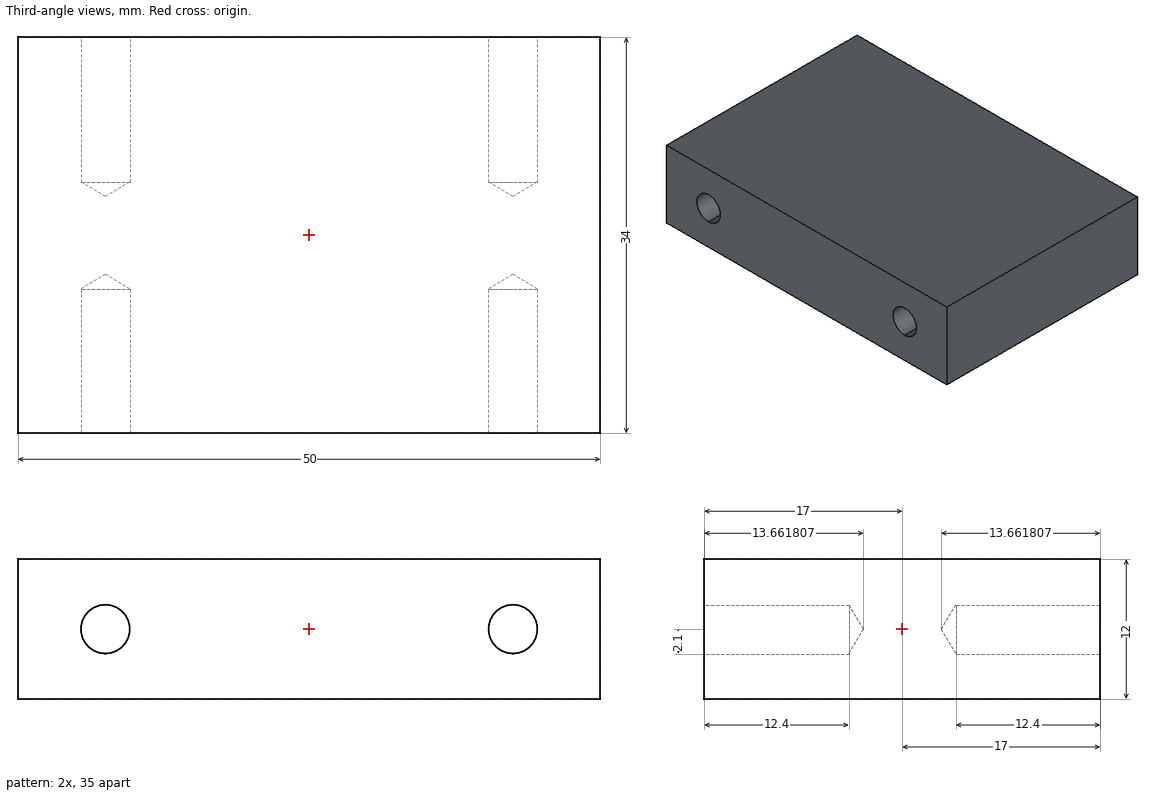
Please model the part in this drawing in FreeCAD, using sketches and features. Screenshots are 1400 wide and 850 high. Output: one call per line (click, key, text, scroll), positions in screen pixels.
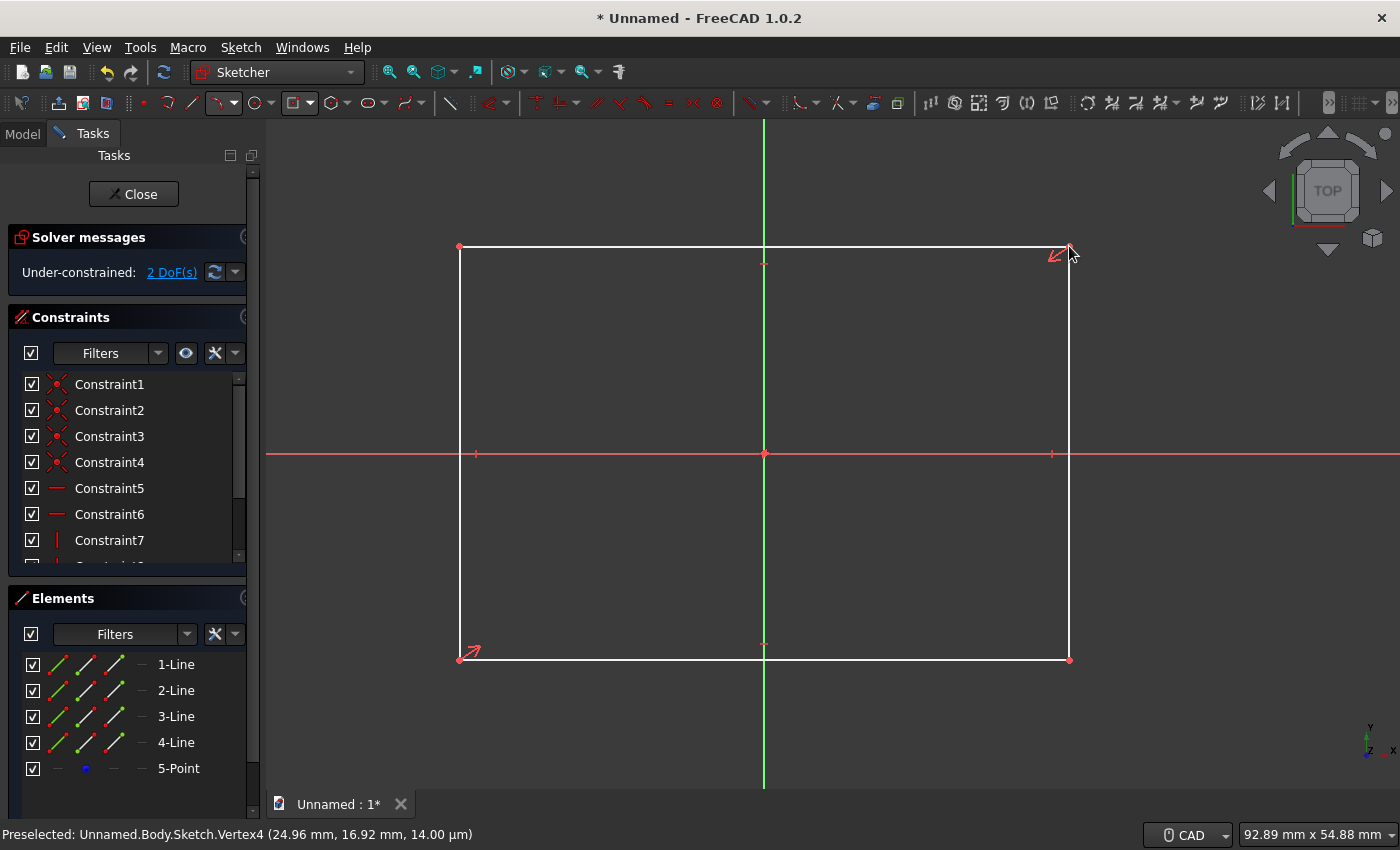
click(642, 660)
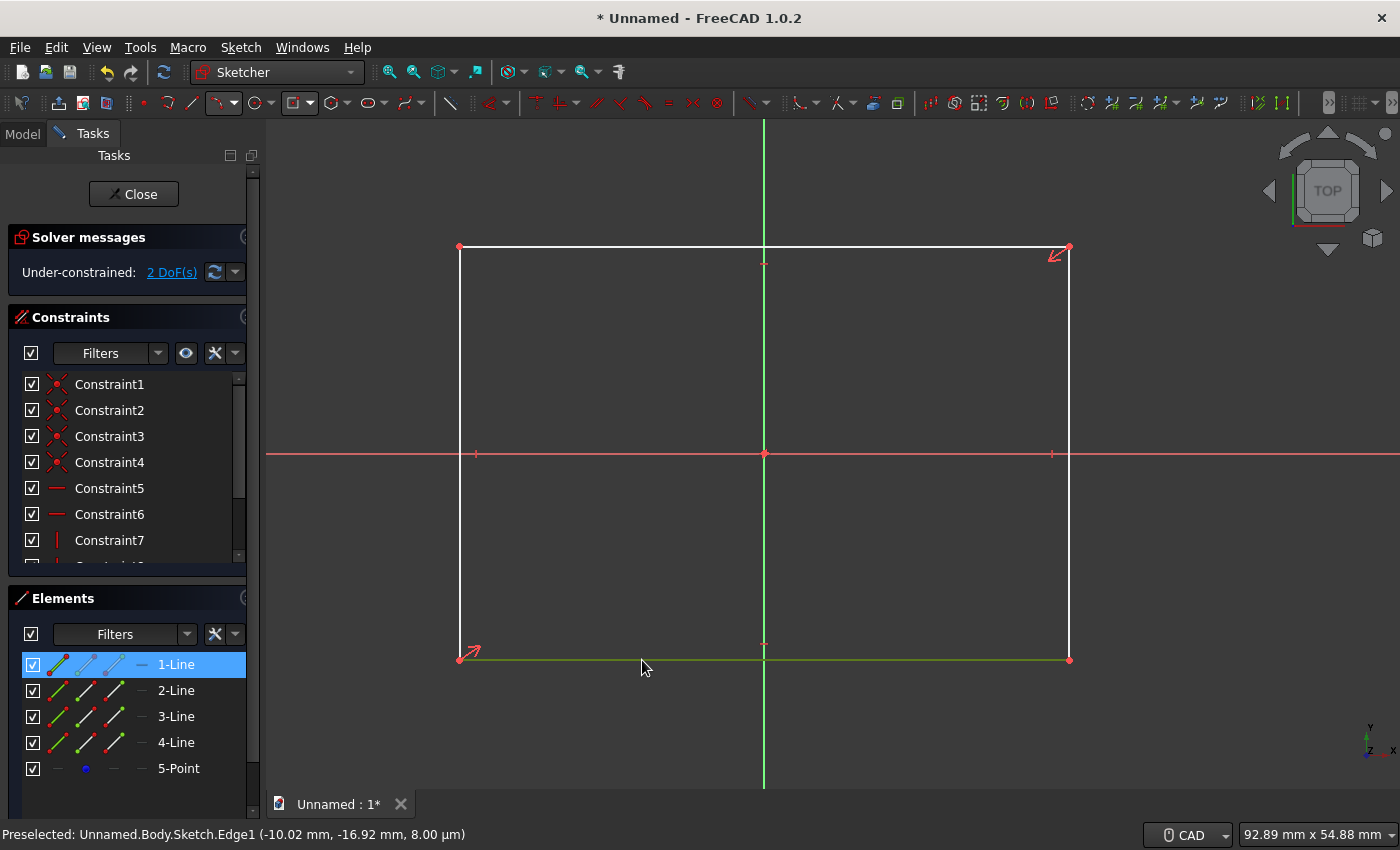
key(l)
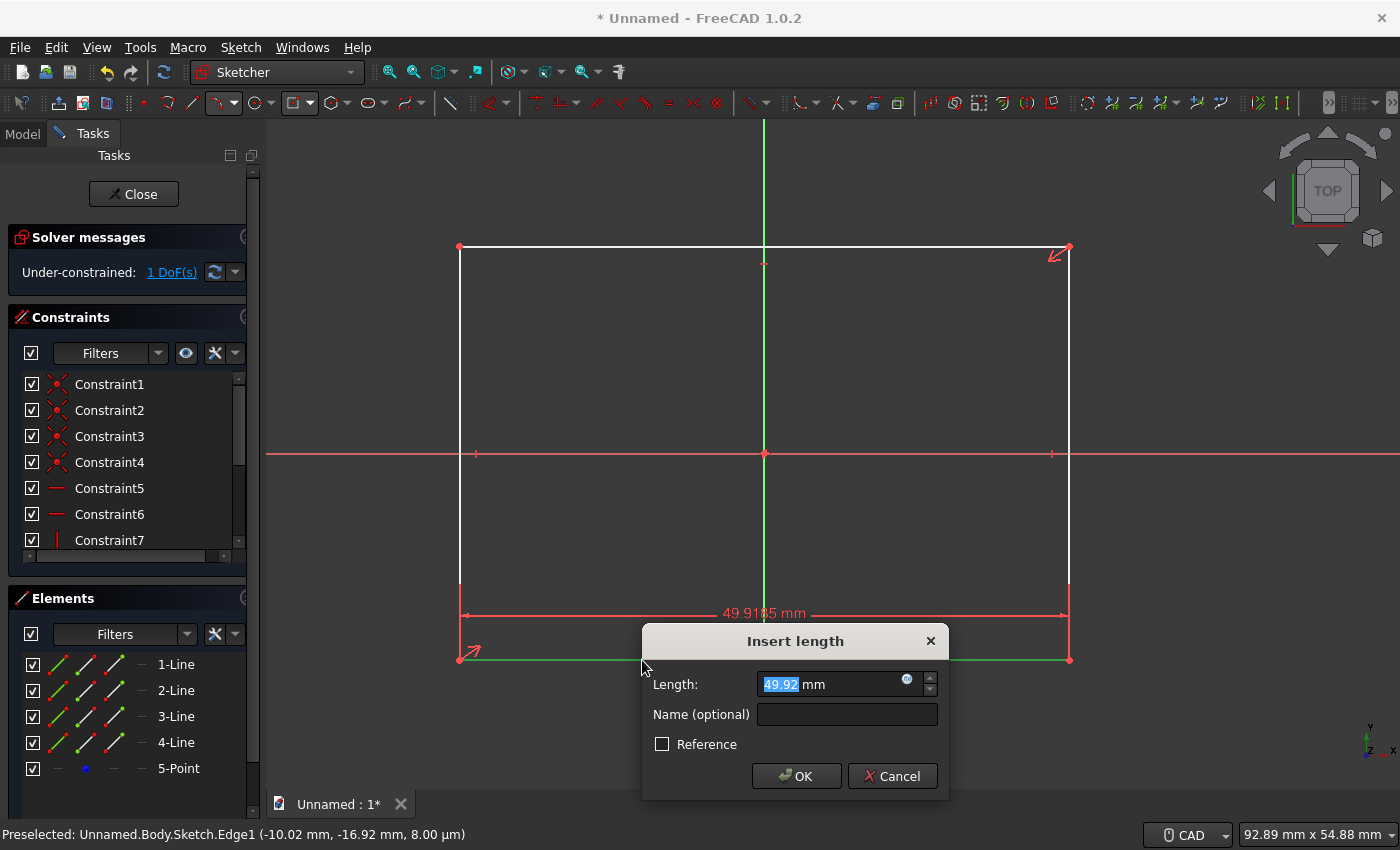
text(50)
key(Return)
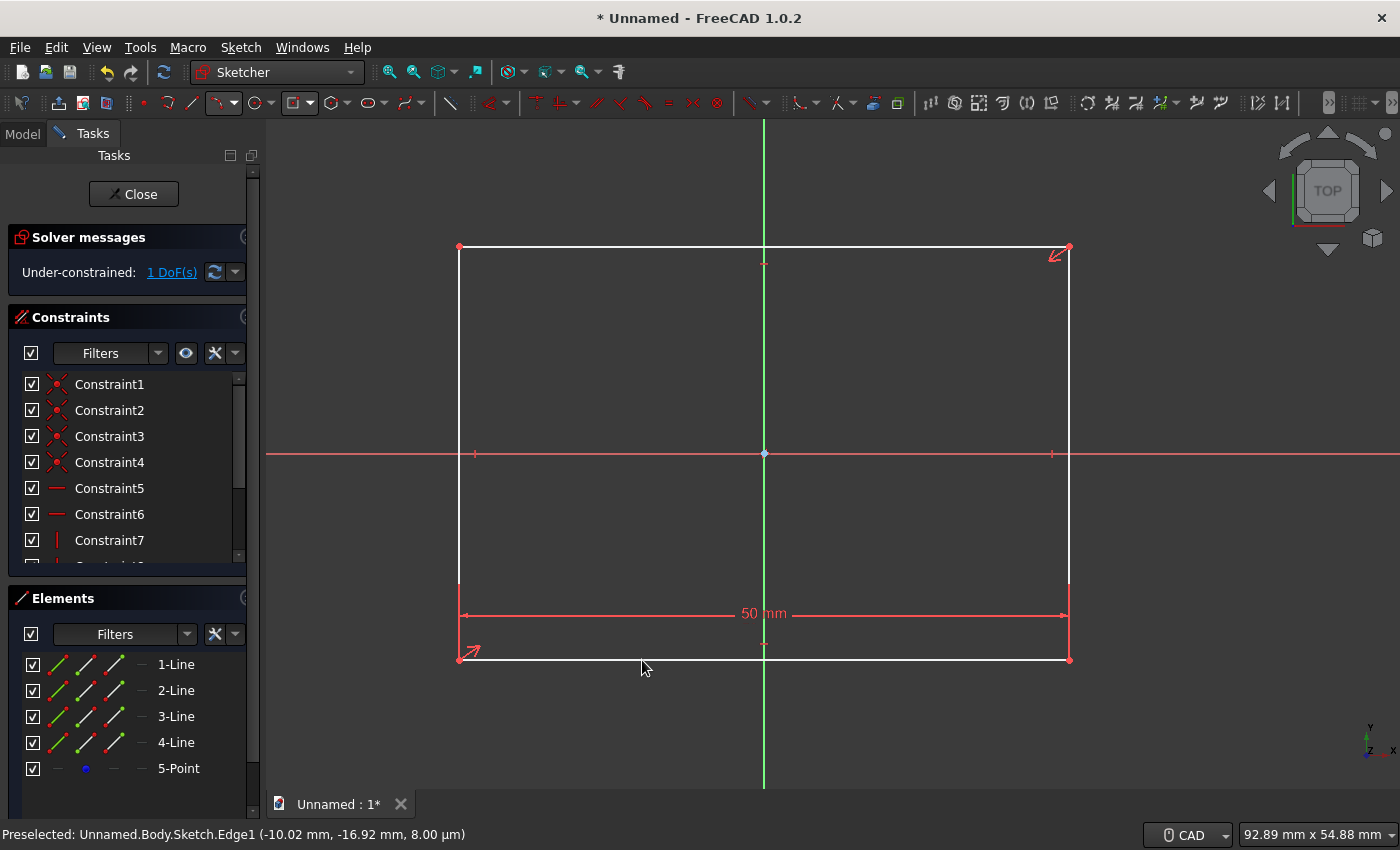
click(1069, 536)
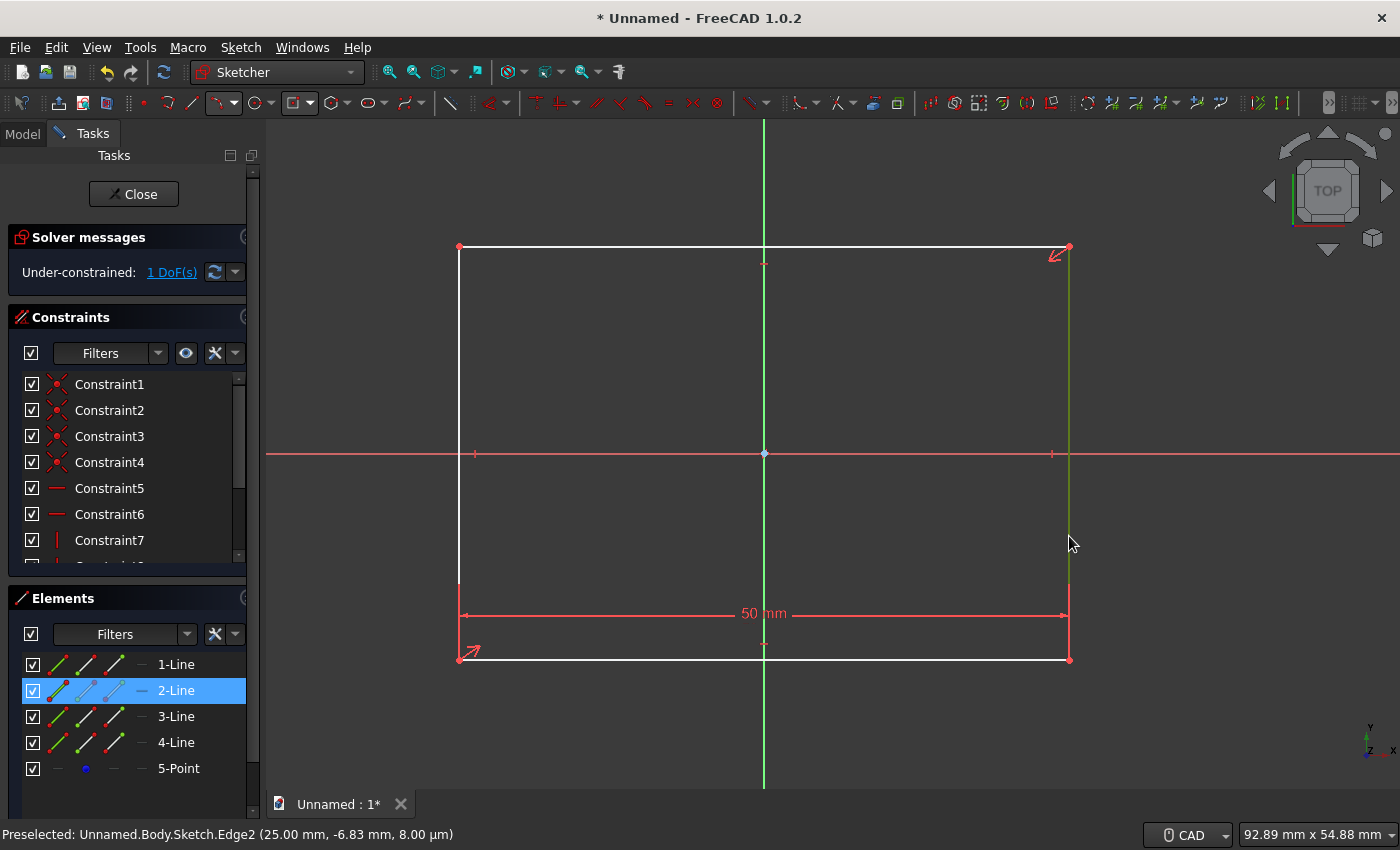
key(i)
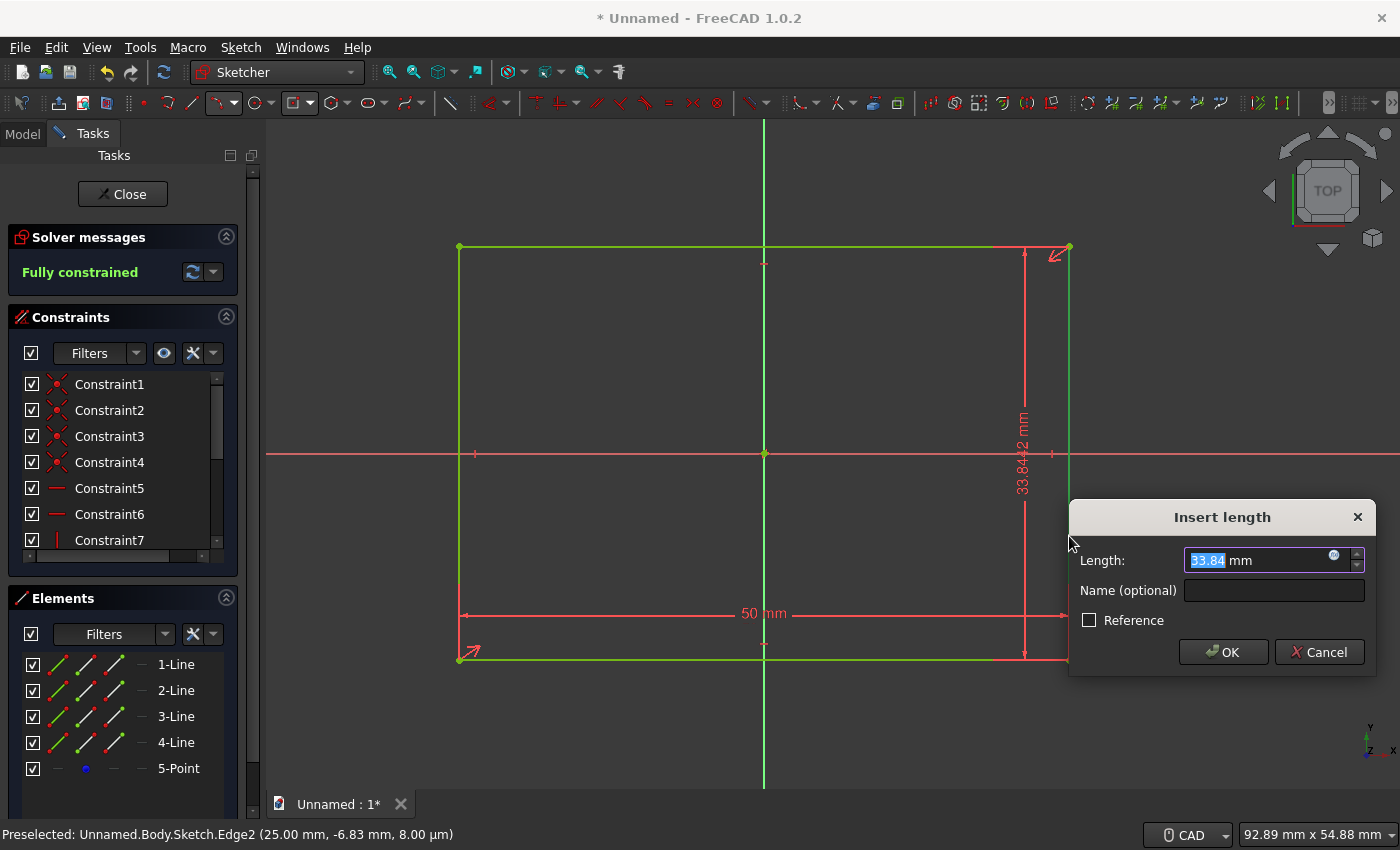
text(34)
key(Return)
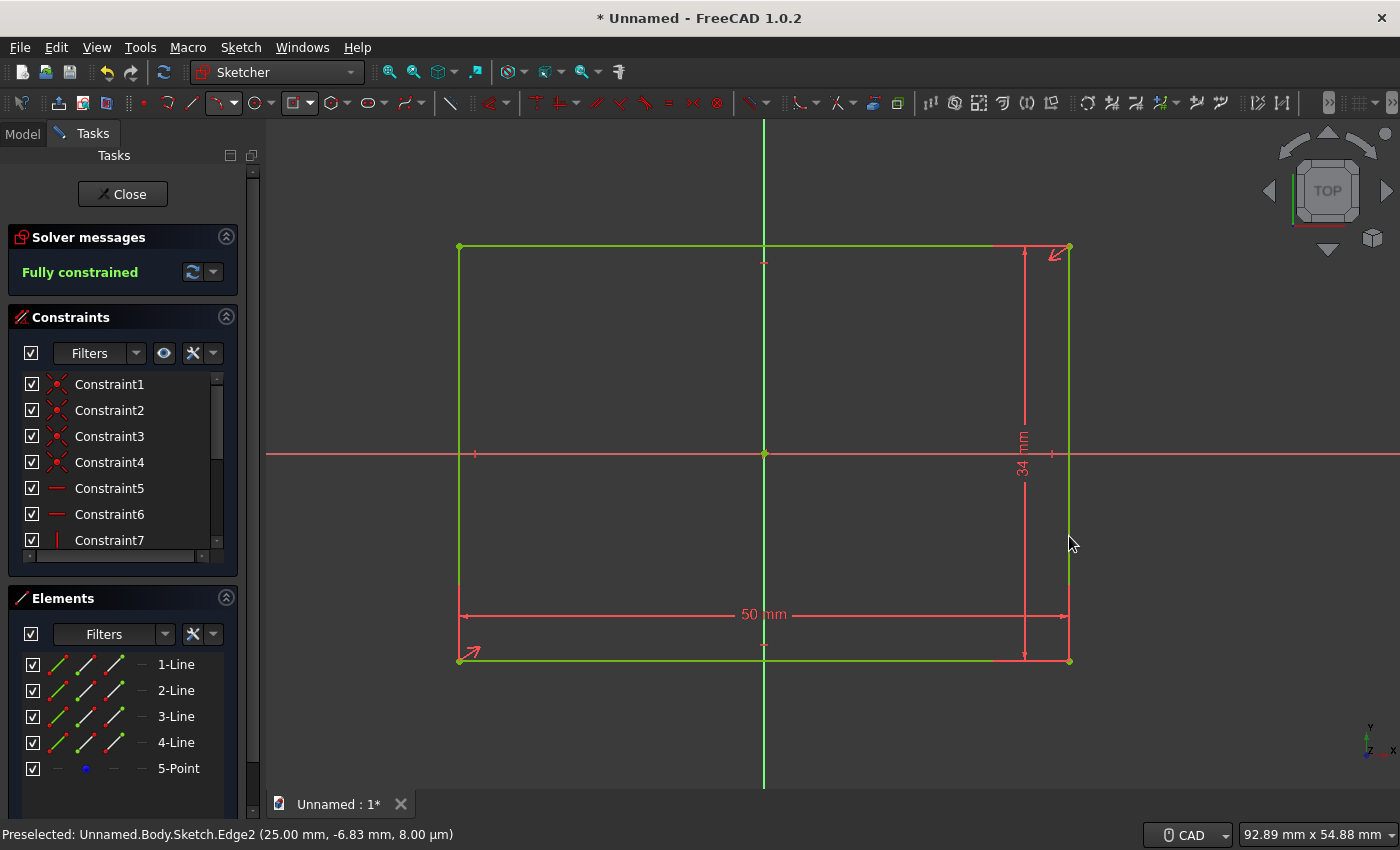
click(123, 194)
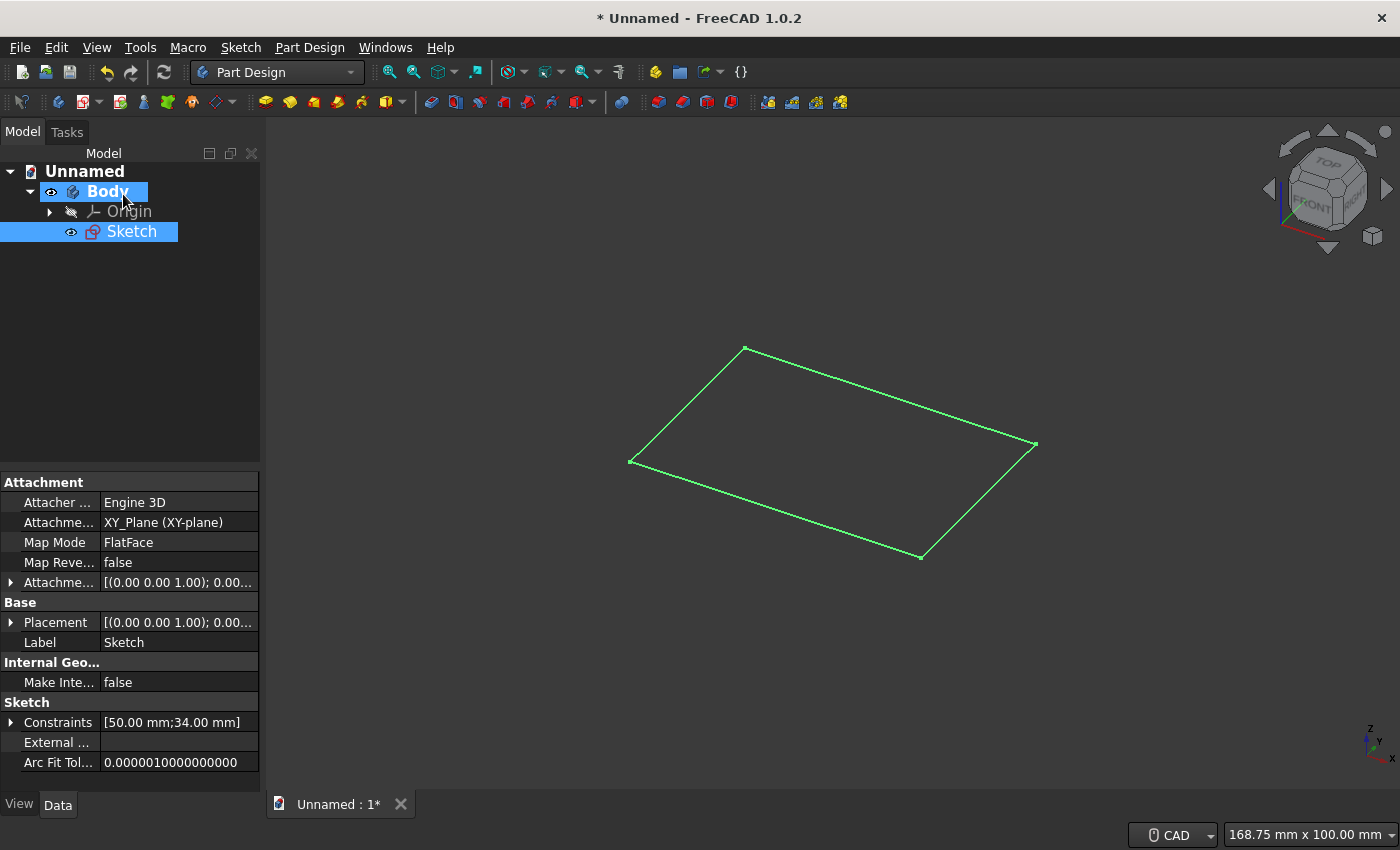
click(266, 102)